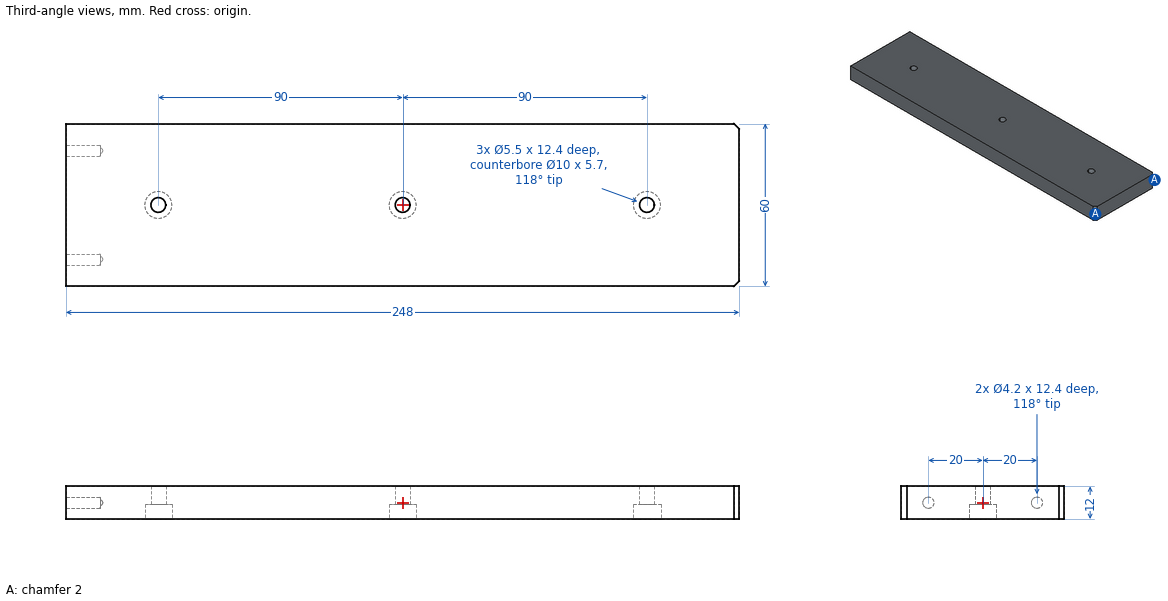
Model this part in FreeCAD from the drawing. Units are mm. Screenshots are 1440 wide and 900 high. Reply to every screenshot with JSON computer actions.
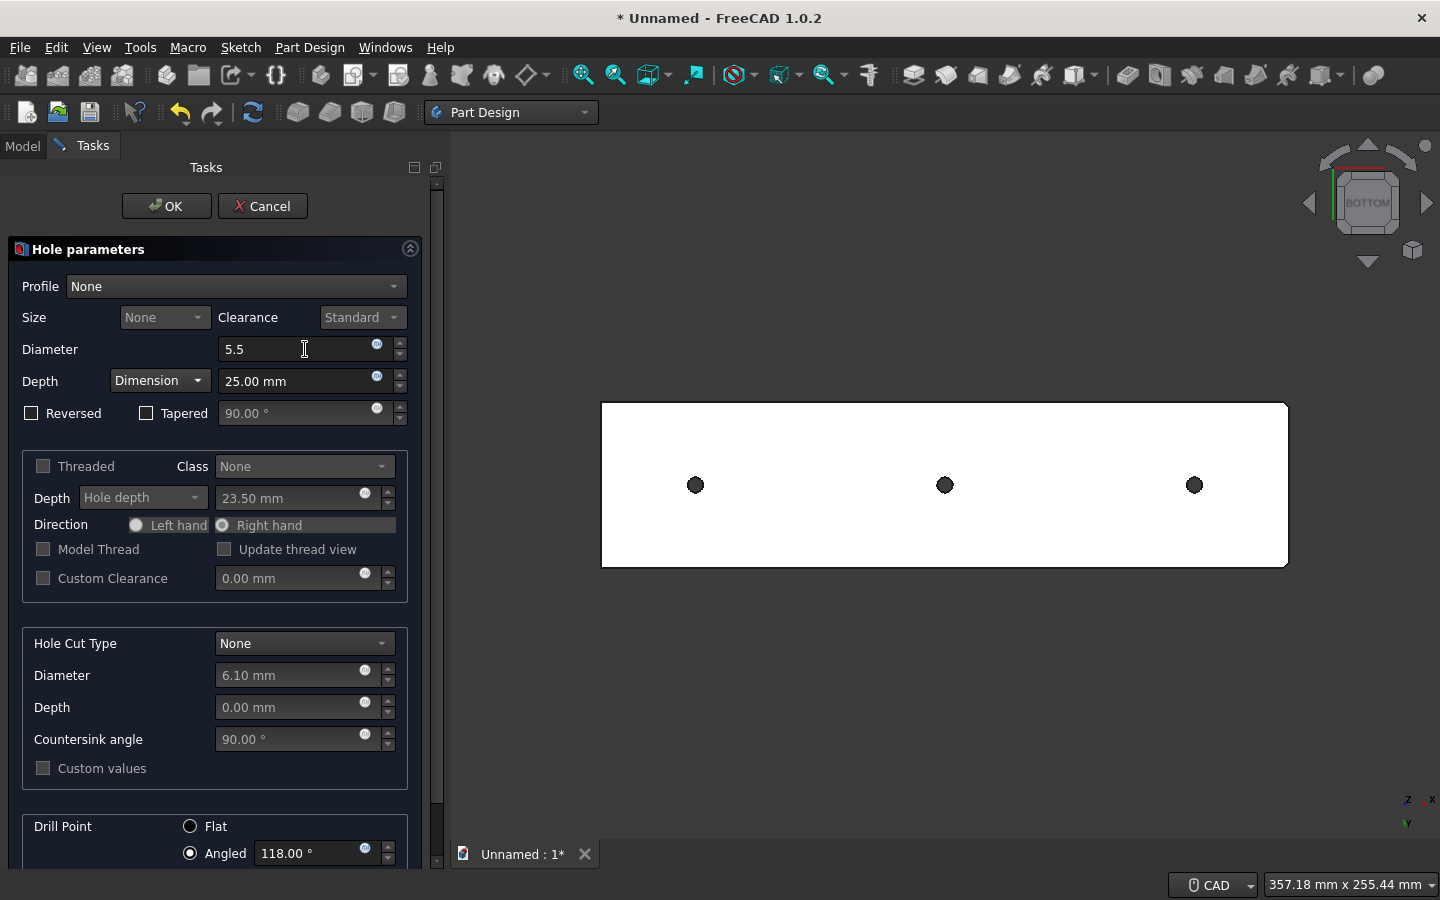
{"action": "triple_click", "coordinate": [305, 381]}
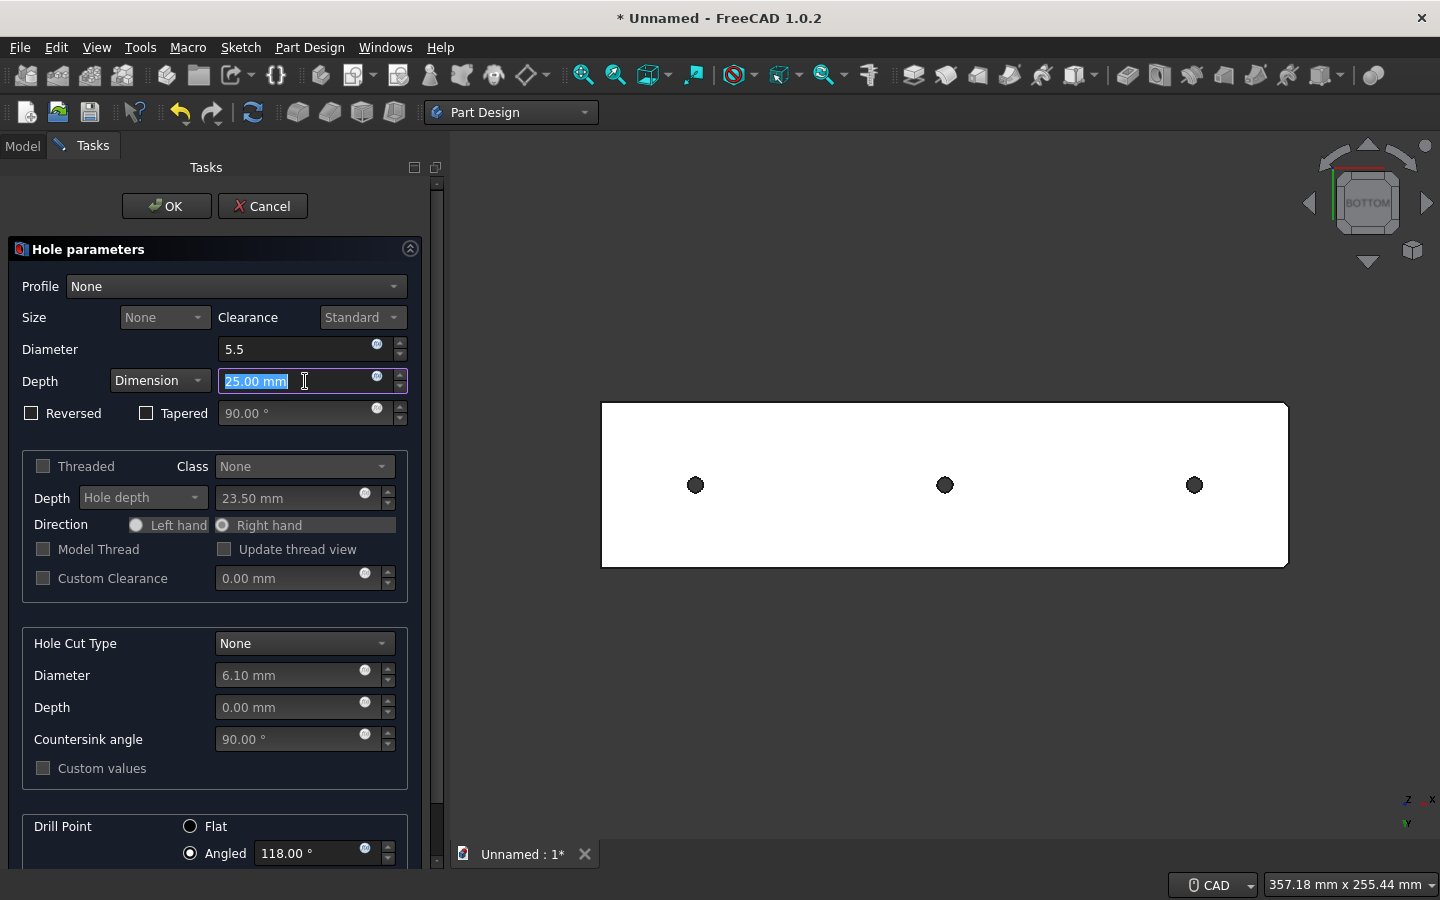
{"action": "type", "text": "12.4"}
{"action": "key", "text": "Tab"}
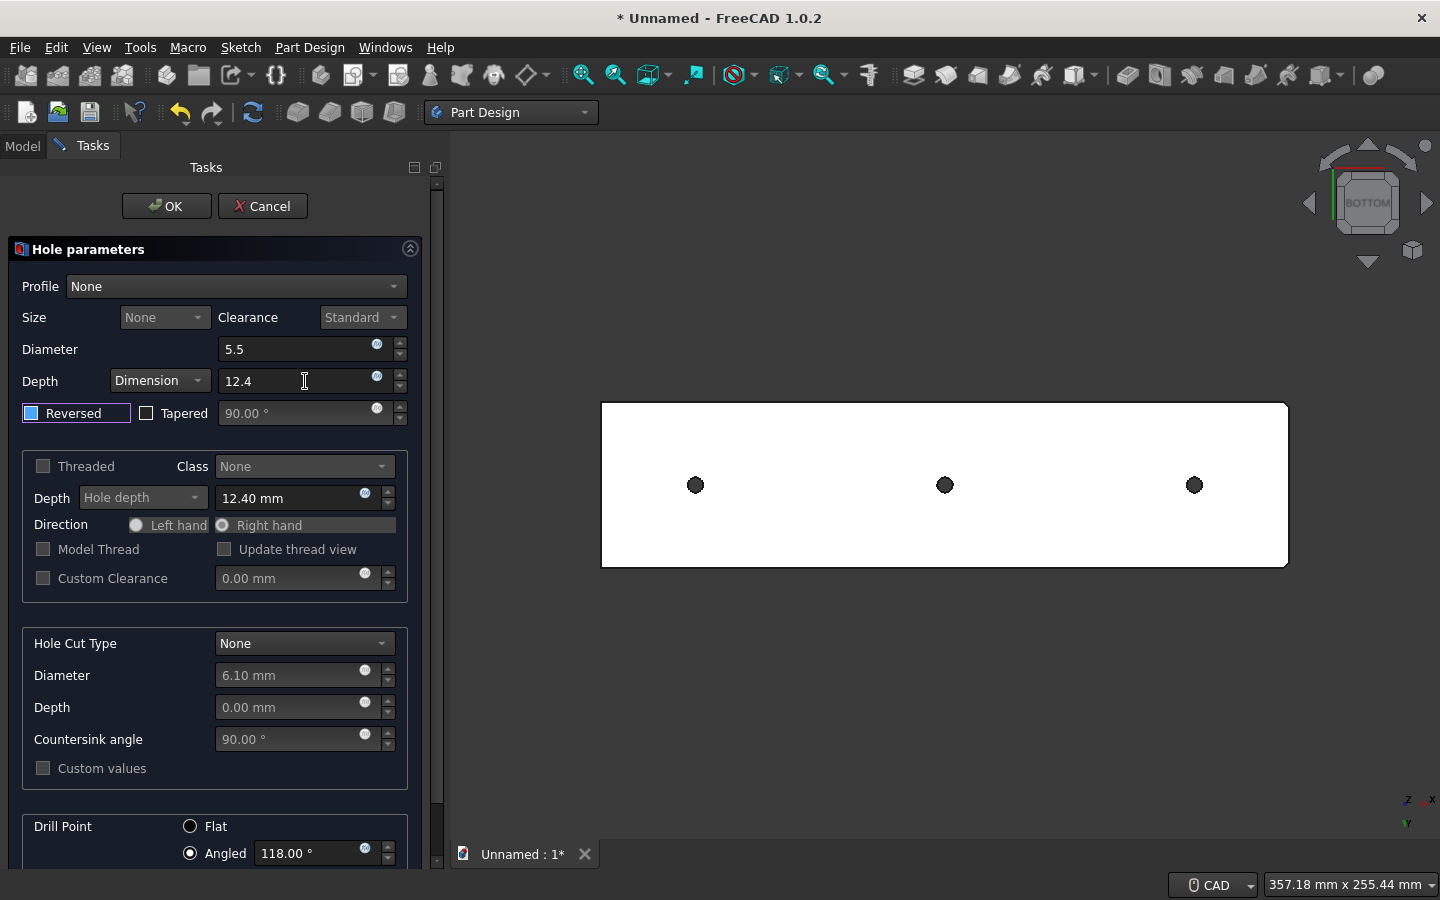
{"action": "left_click", "coordinate": [306, 644]}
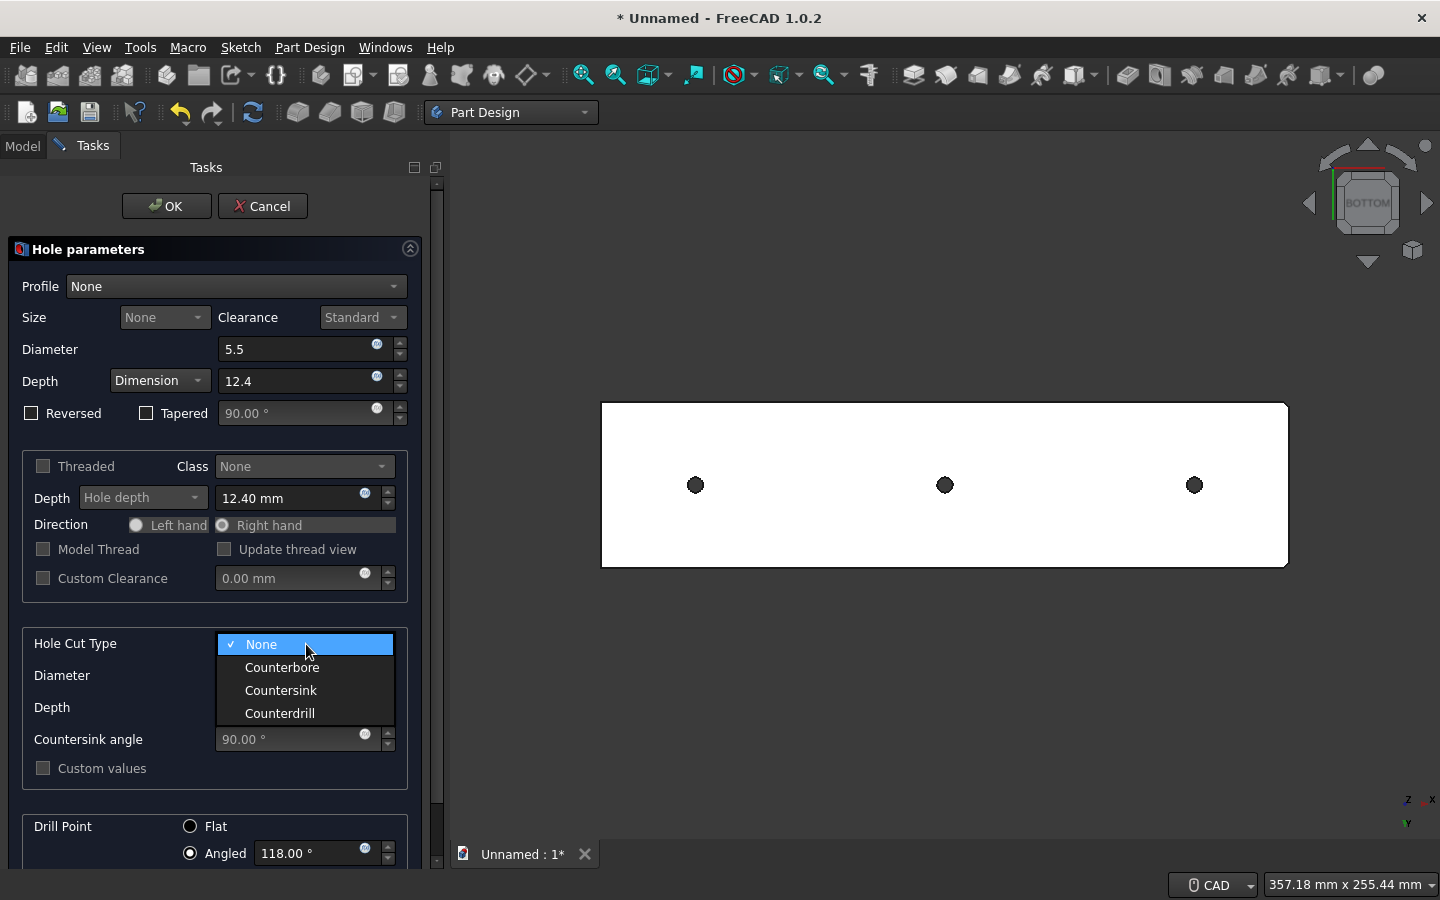
{"action": "left_click", "coordinate": [304, 668]}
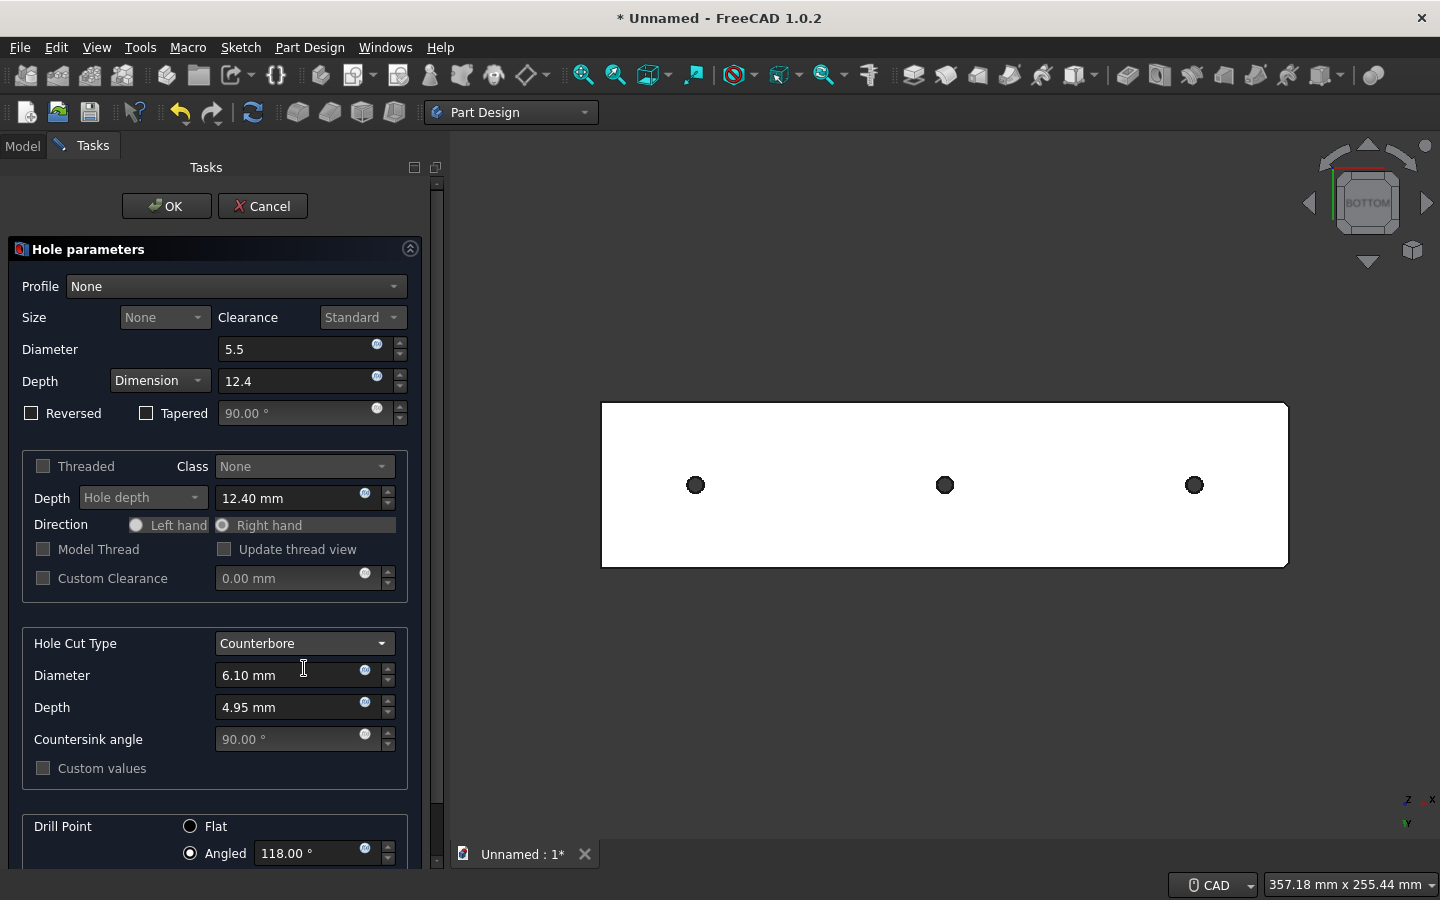
{"action": "triple_click", "coordinate": [298, 675]}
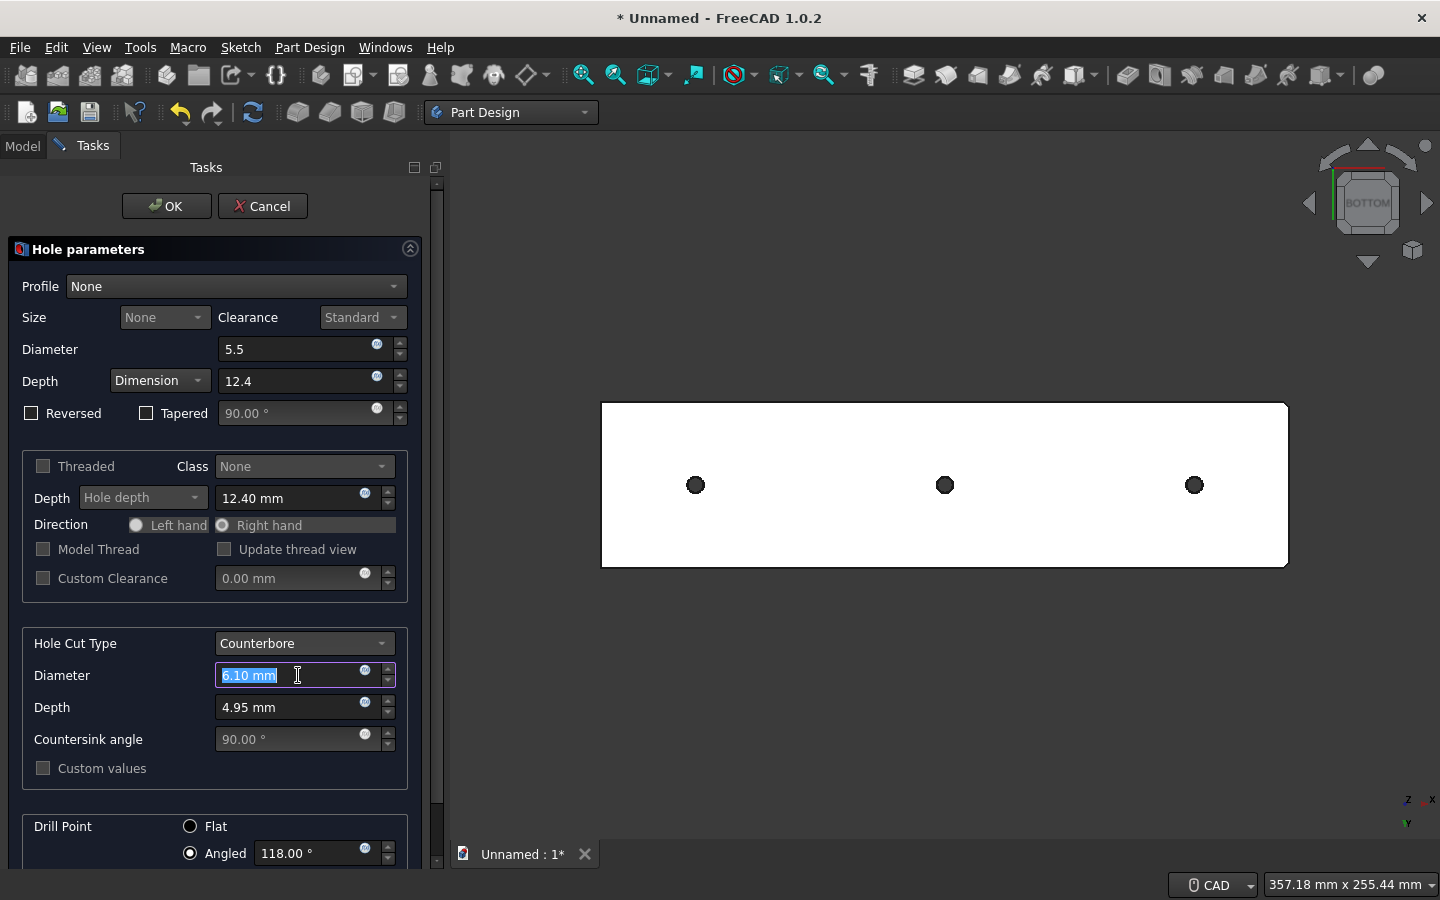
{"action": "type", "text": "10"}
{"action": "key", "text": "Tab"}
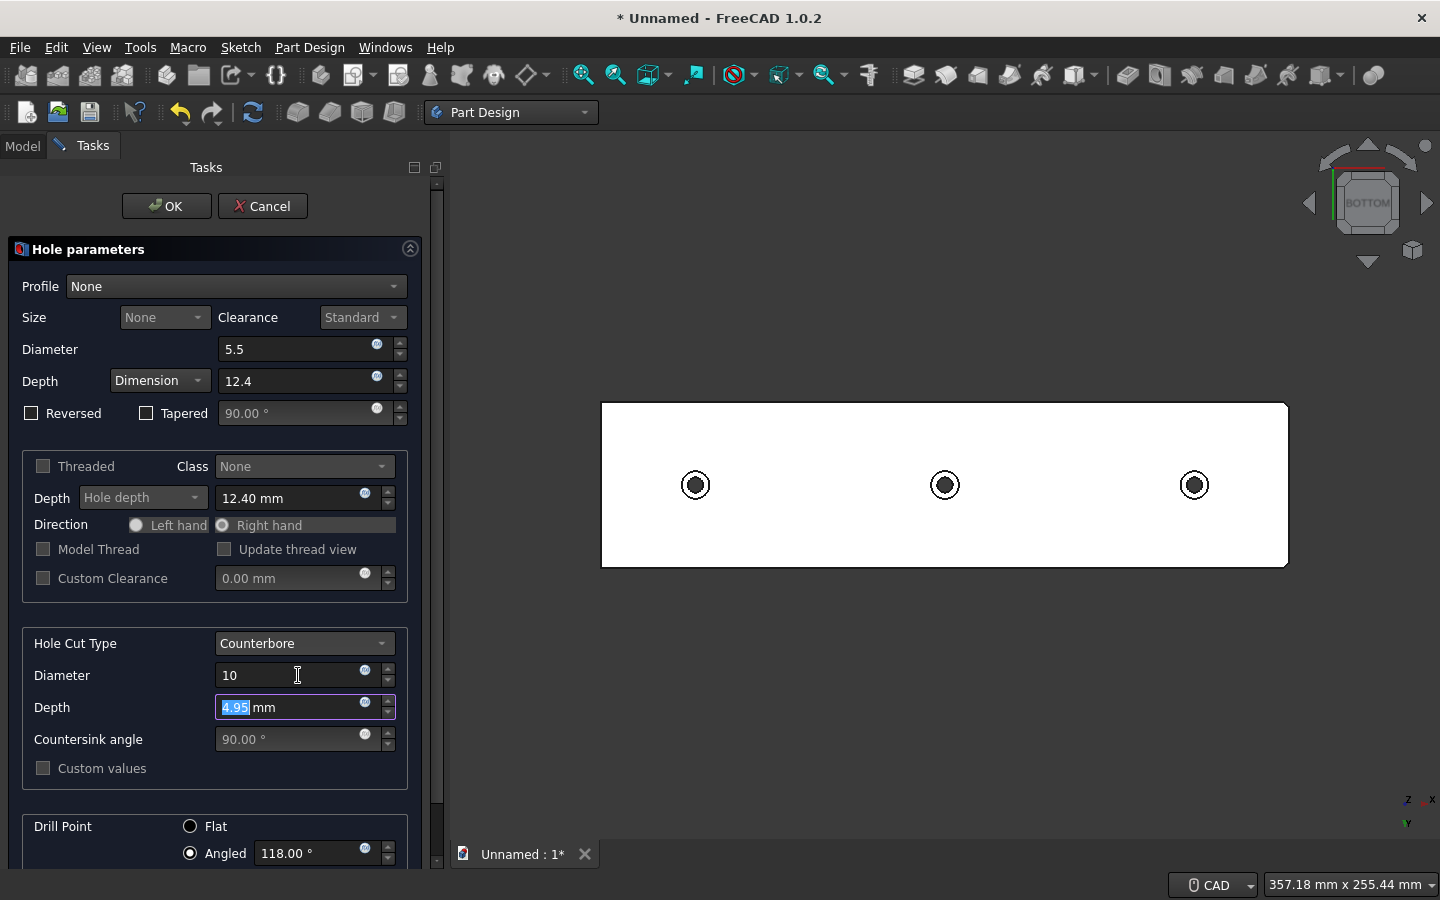
{"action": "type", "text": "5.7"}
{"action": "key", "text": "Tab"}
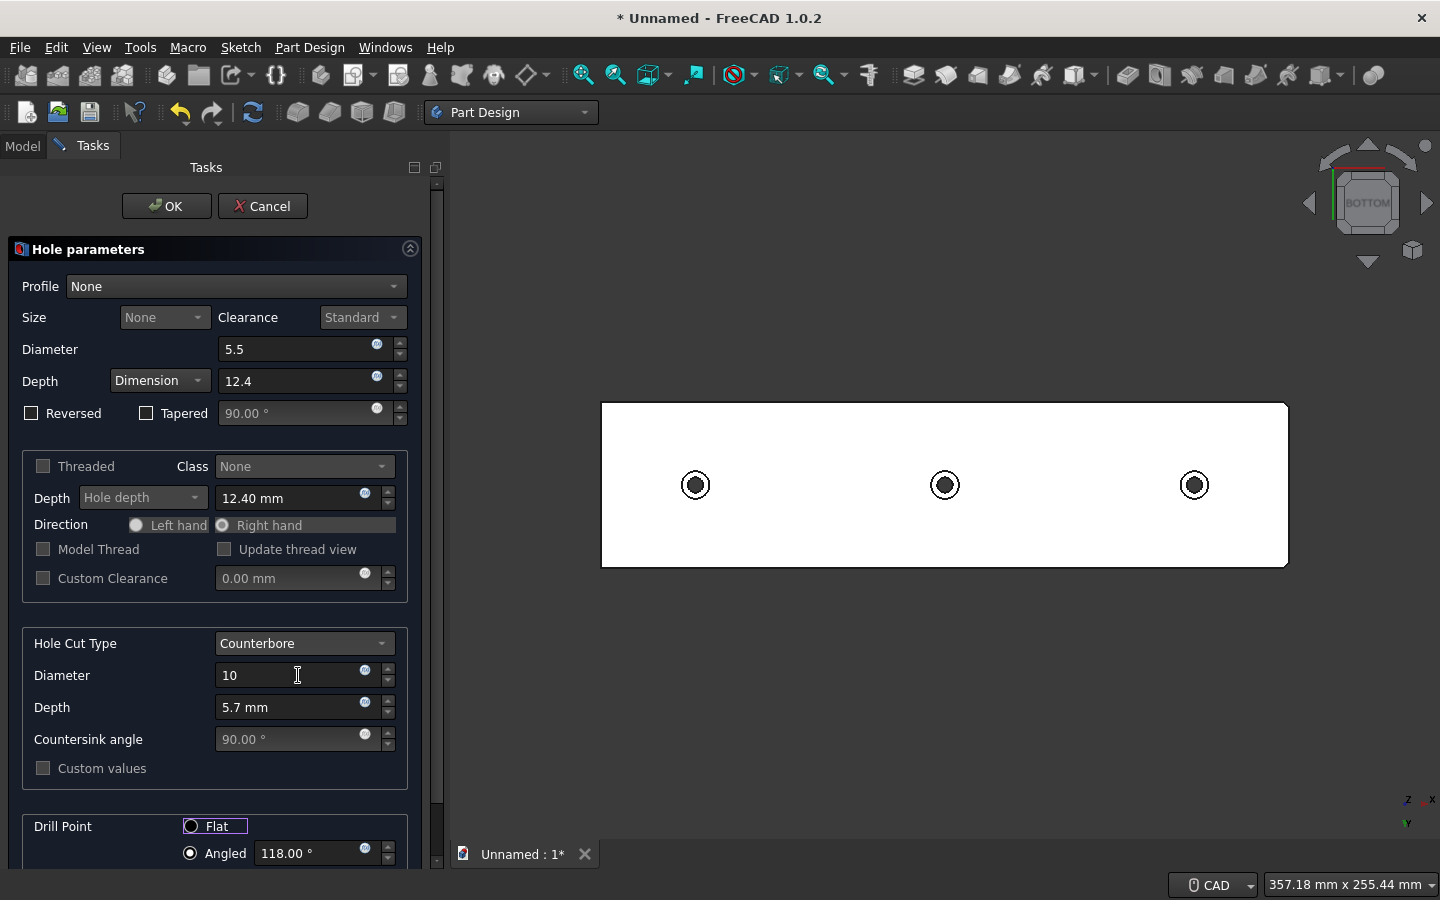
{"action": "left_click", "coordinate": [167, 206]}